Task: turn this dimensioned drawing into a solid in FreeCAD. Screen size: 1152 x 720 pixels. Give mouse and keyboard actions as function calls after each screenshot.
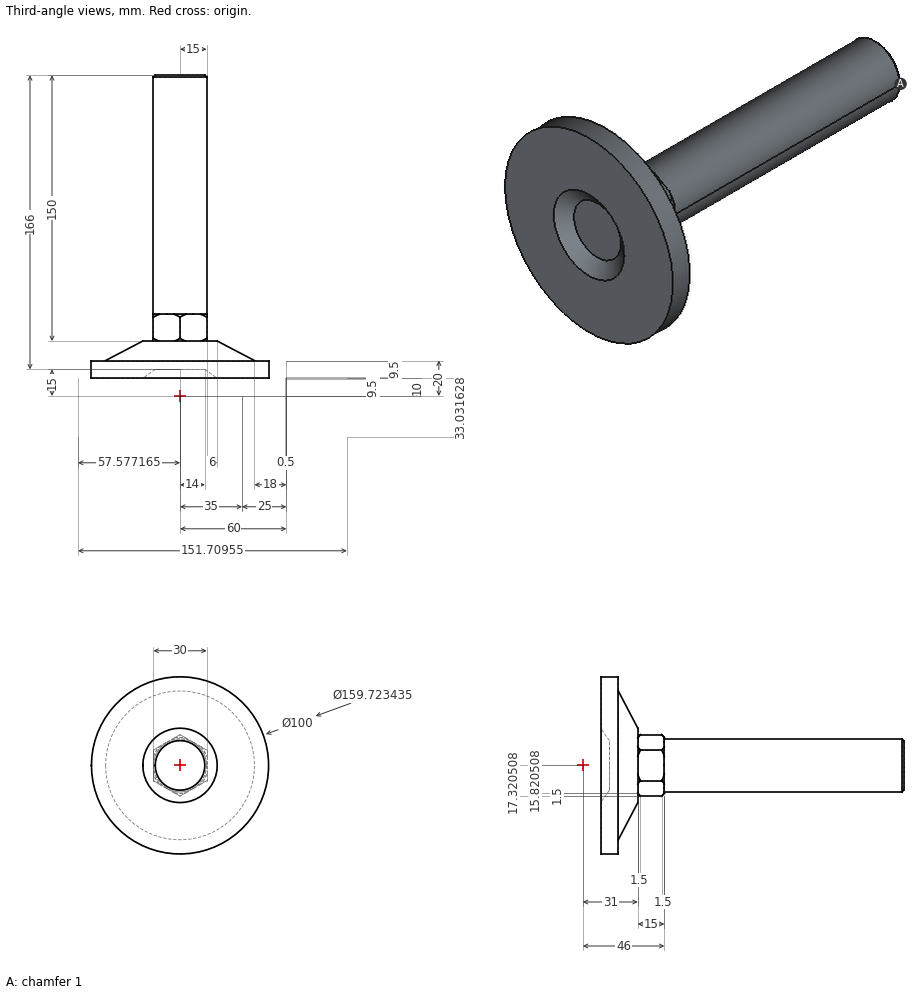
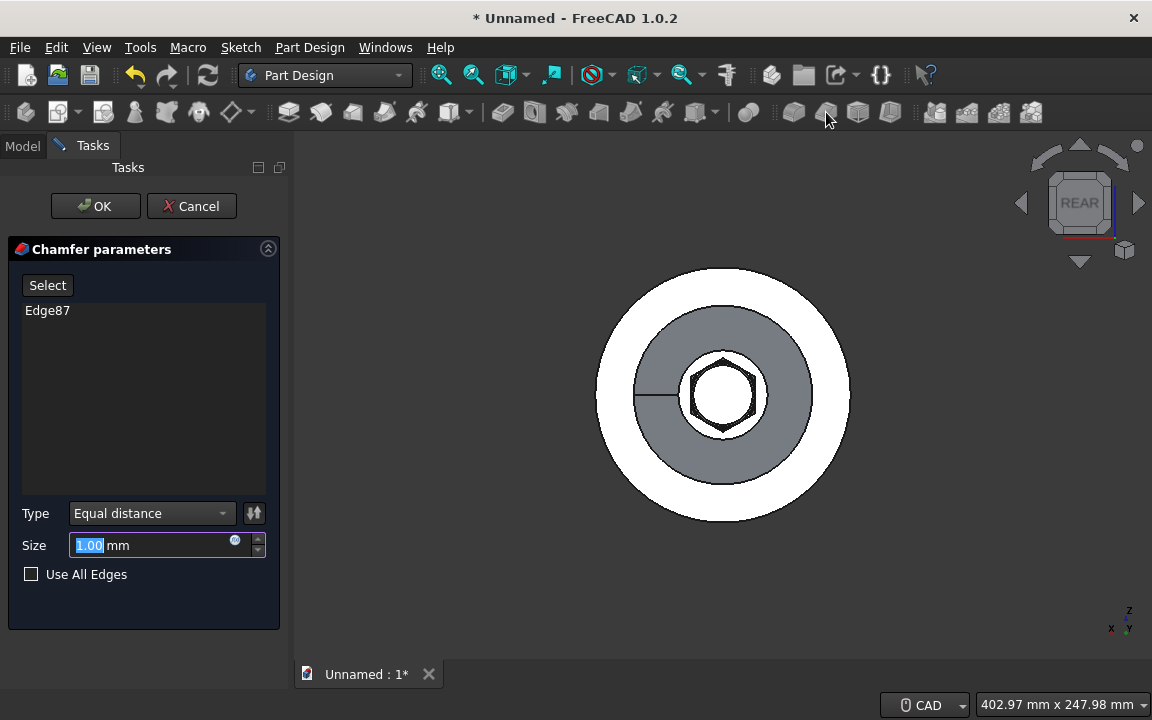
text(1)
key(Tab)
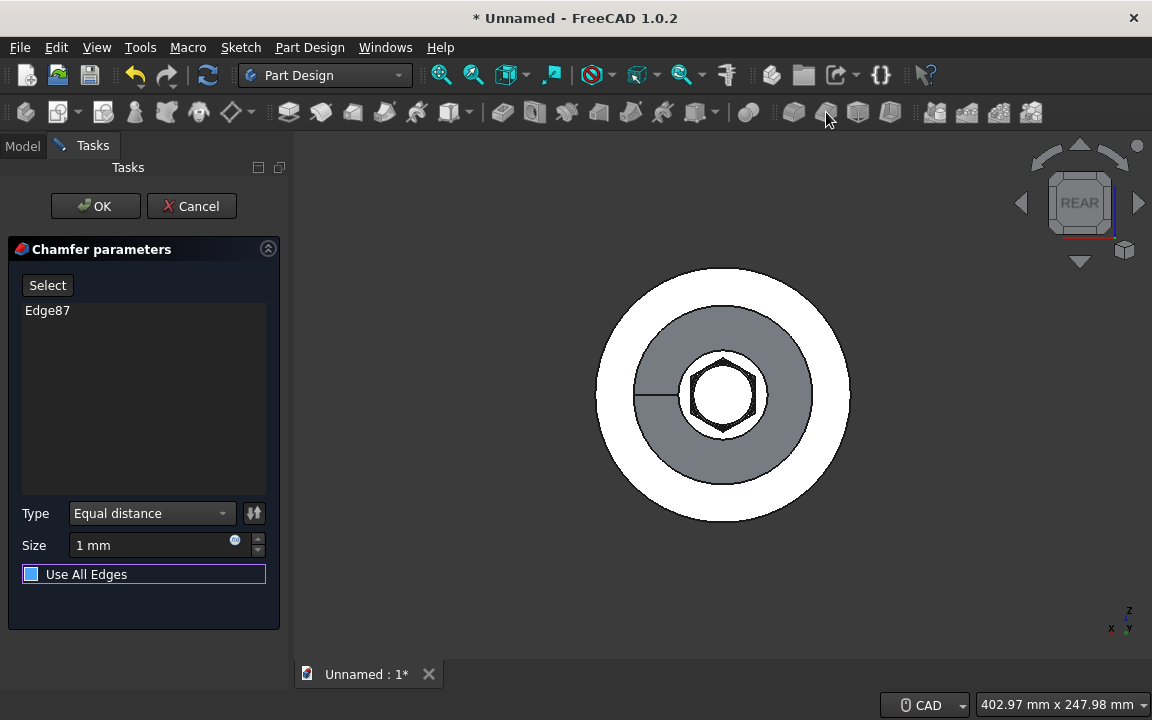
click(96, 206)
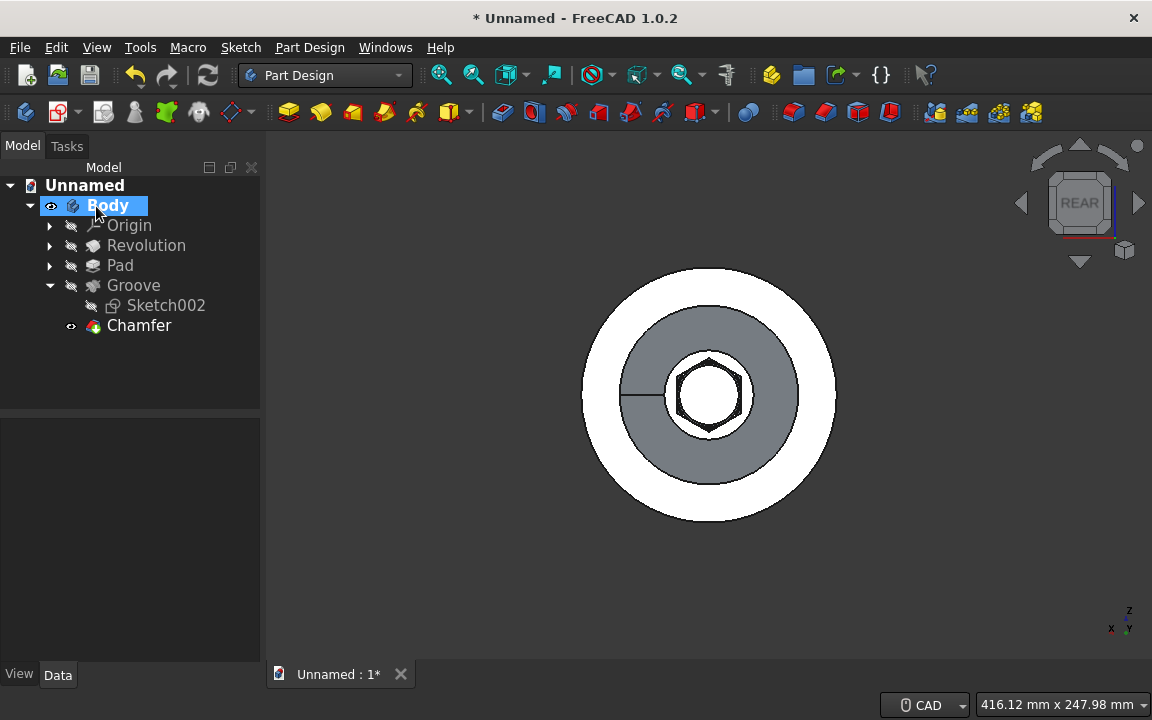
click(599, 394)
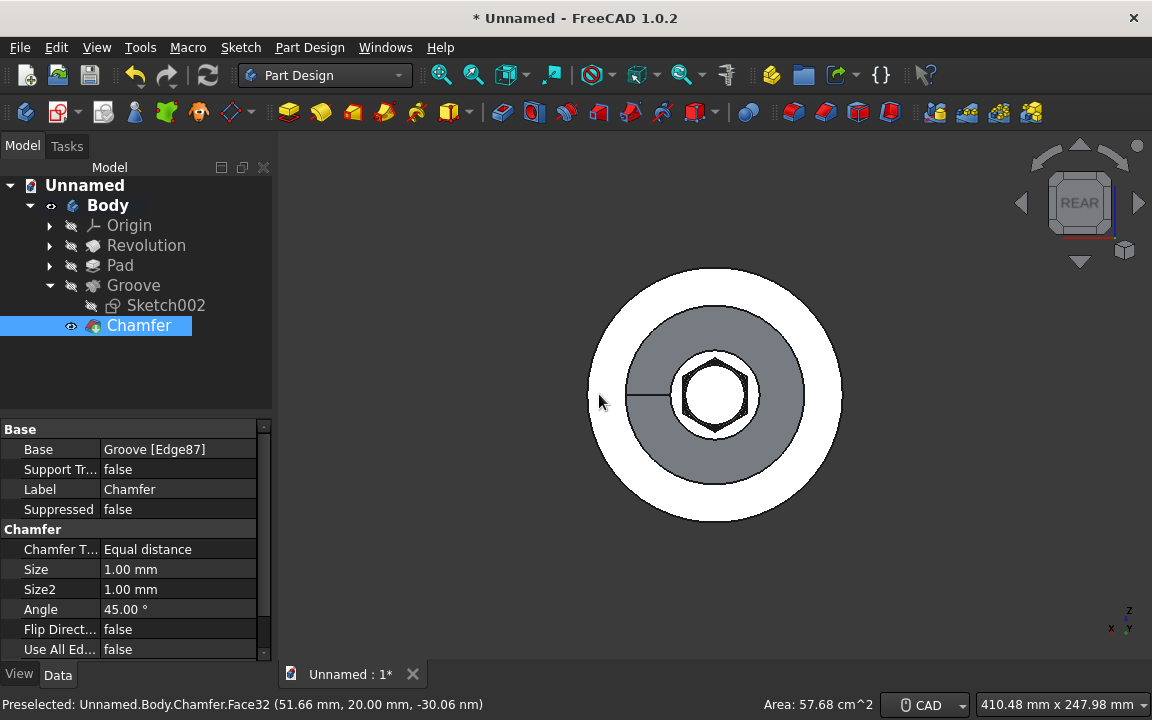
click(58, 112)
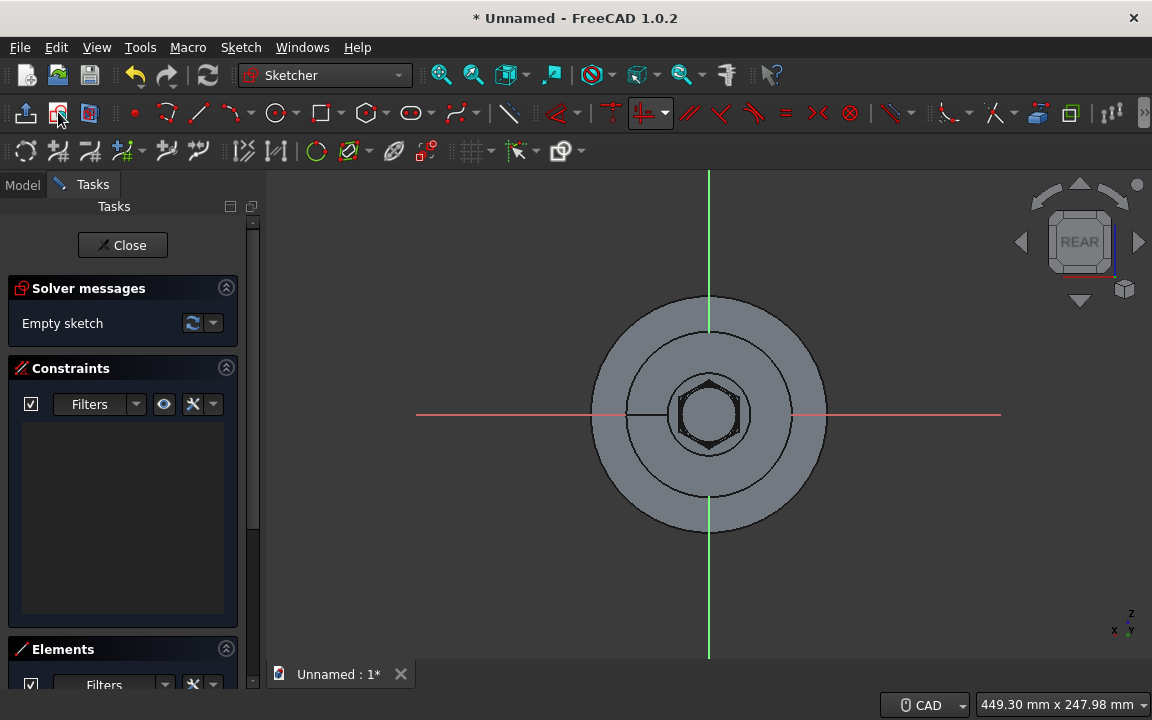
click(276, 114)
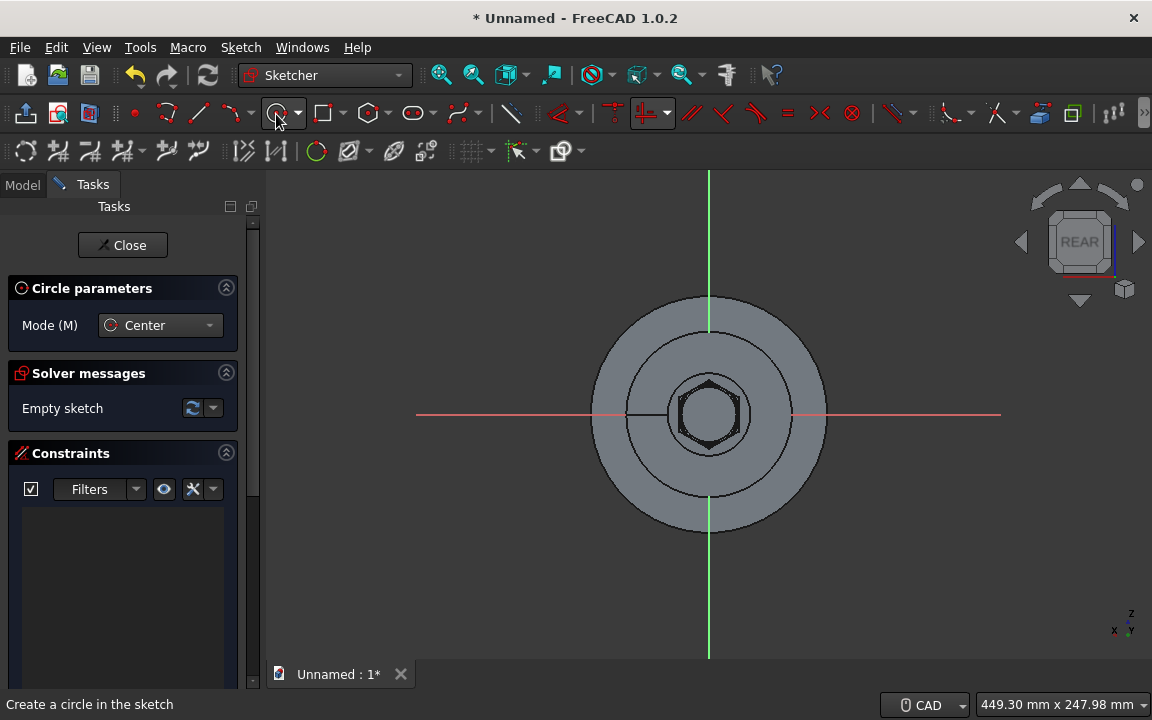
click(709, 415)
move(820, 303)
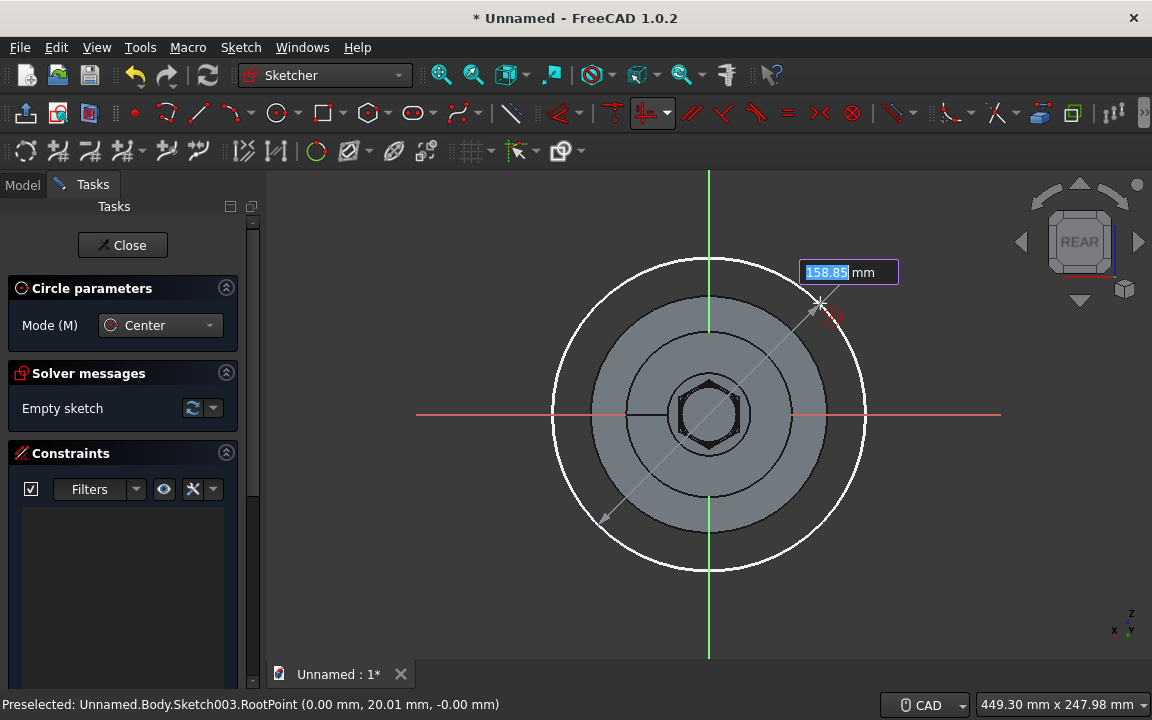
text(159.723435)
key(Return)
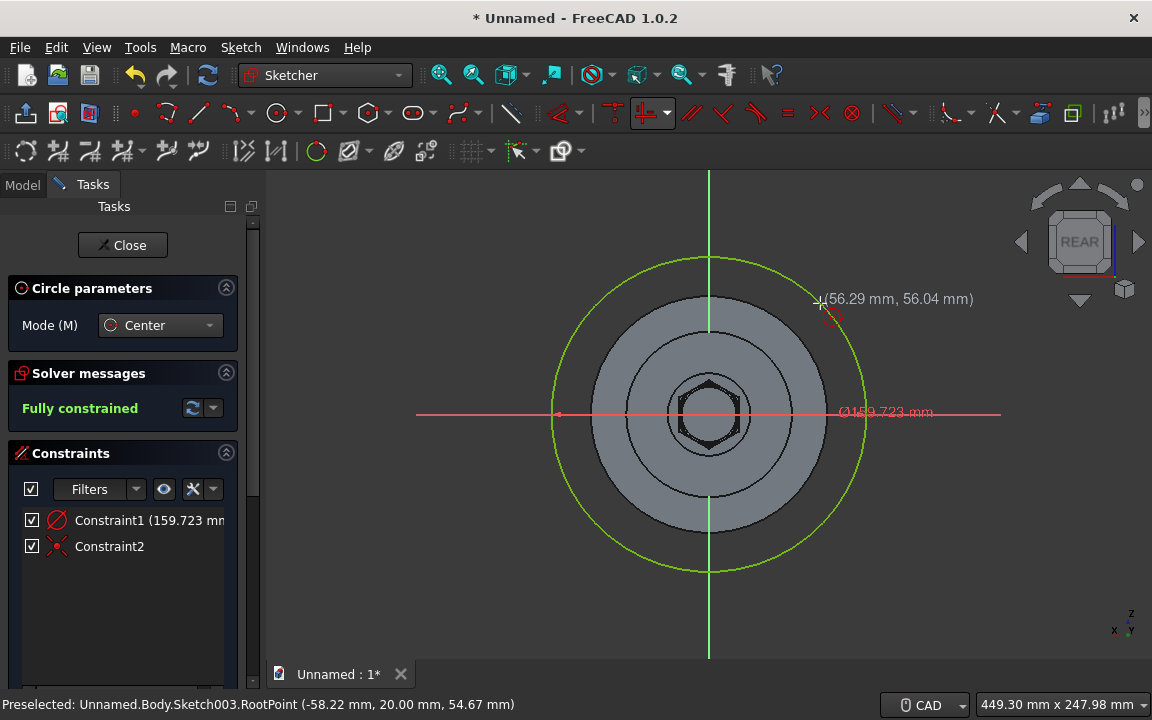
click(709, 415)
move(779, 345)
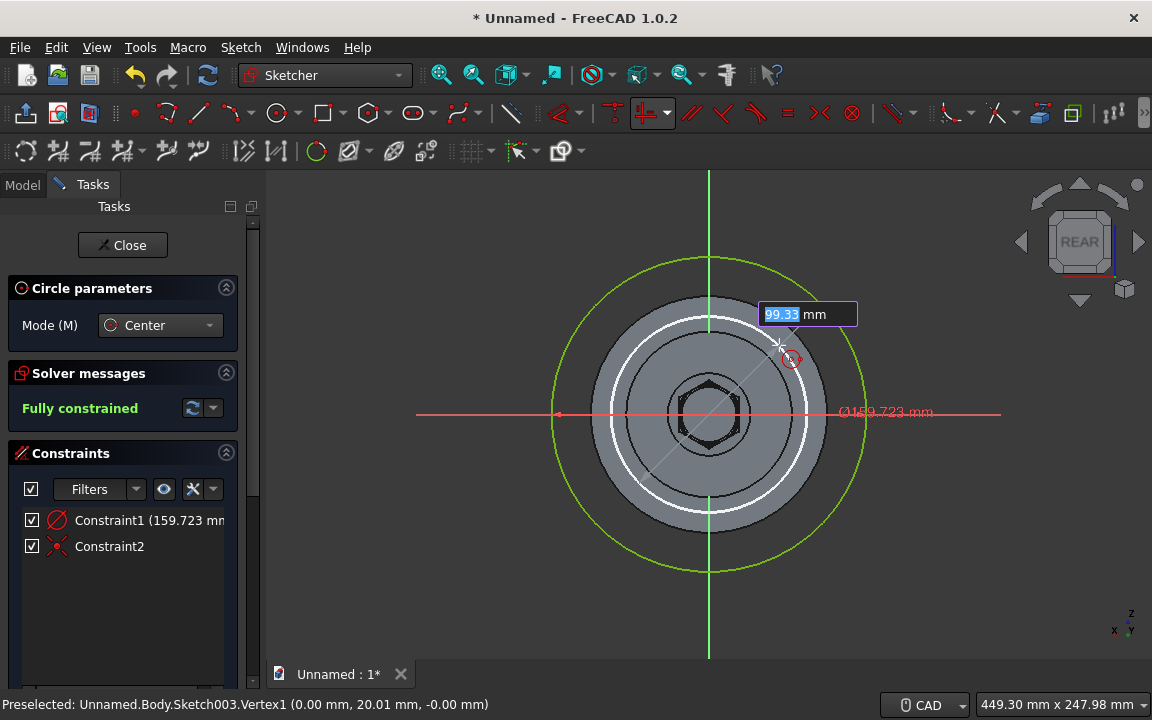
text(100)
key(Return)
key(Escape)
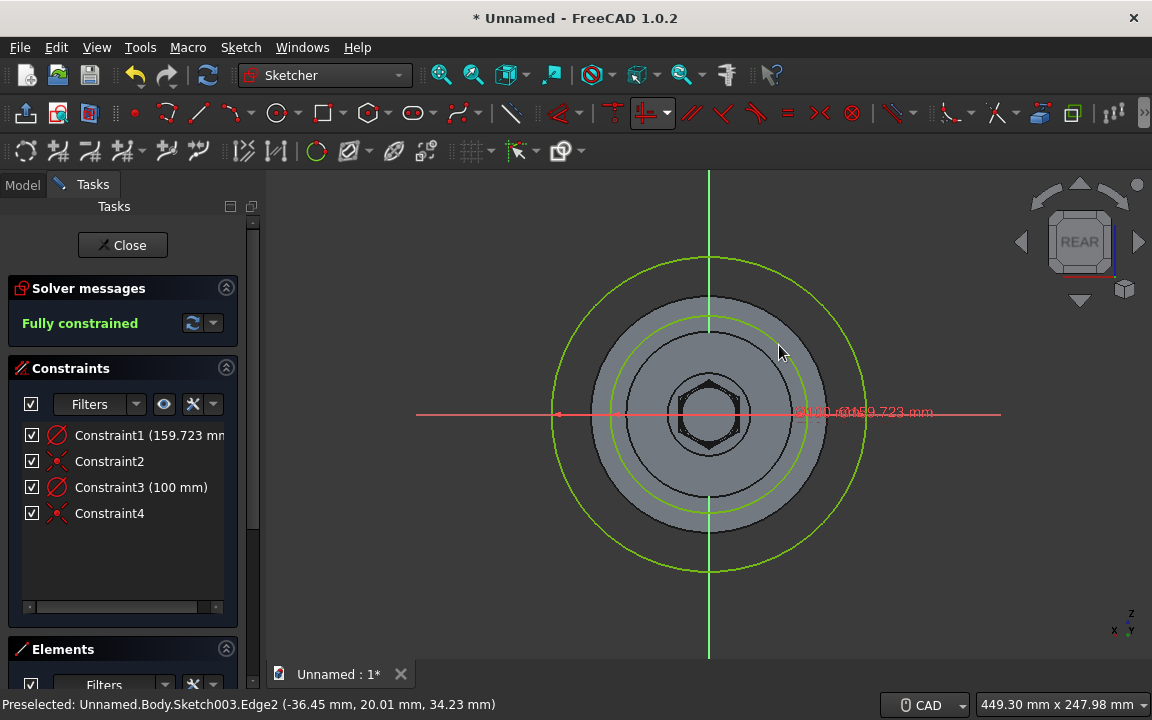
click(123, 245)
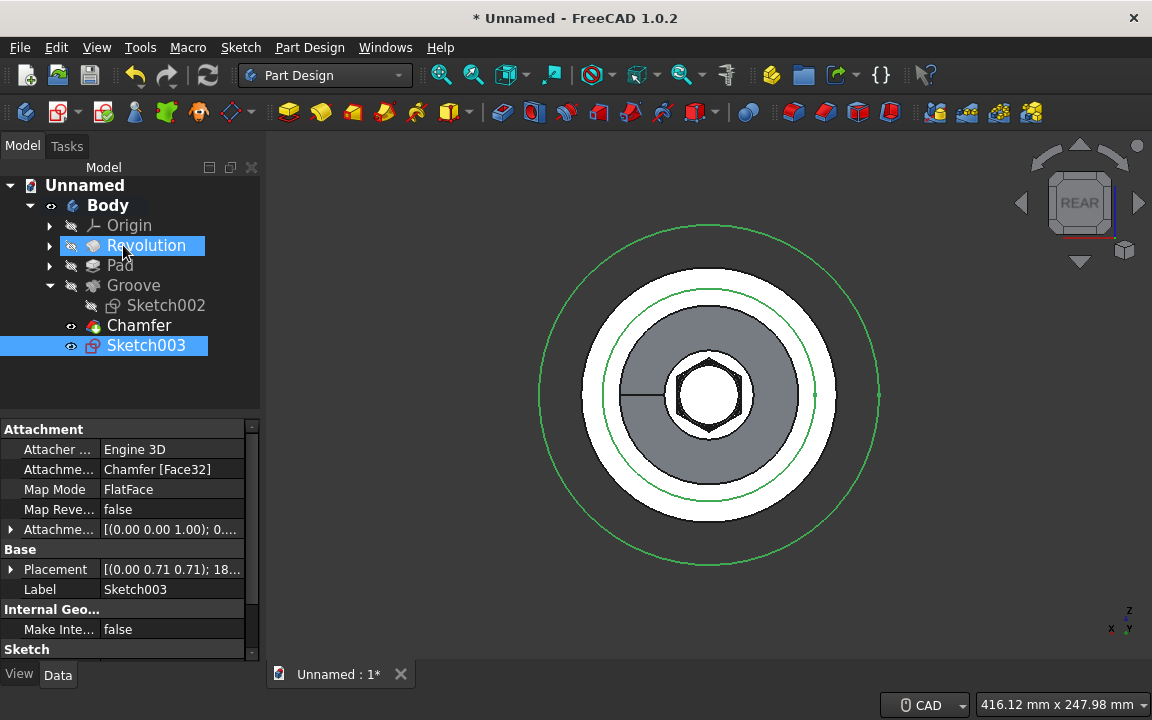
click(504, 112)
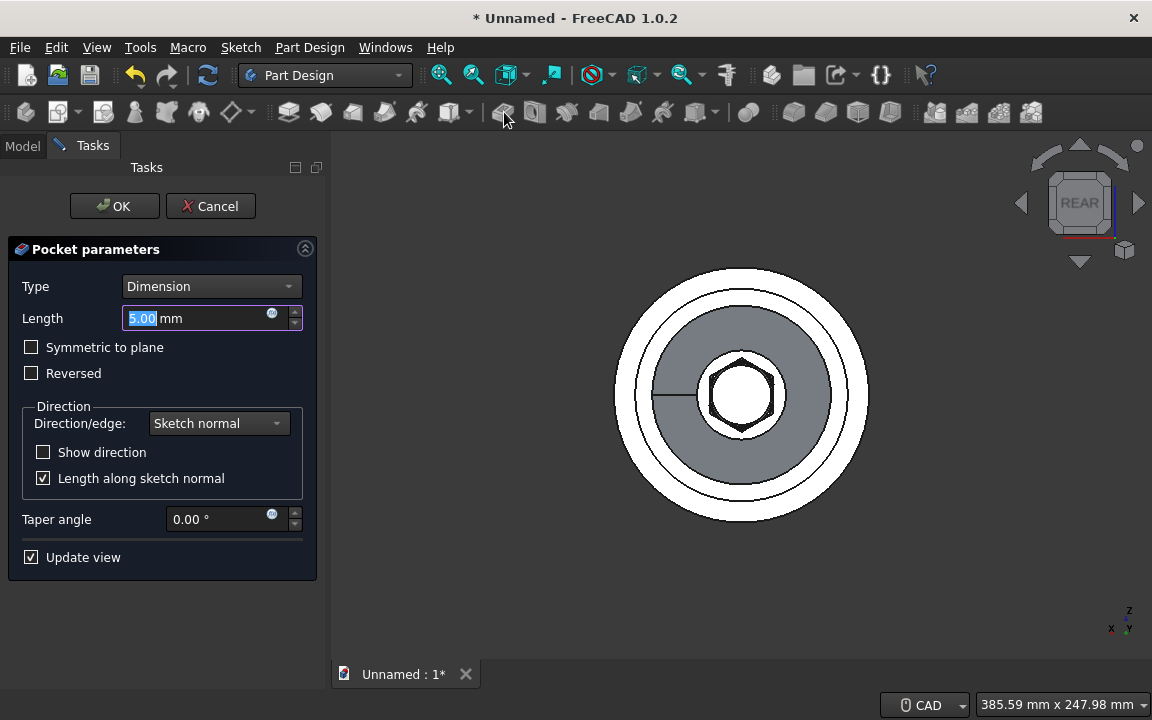
click(212, 286)